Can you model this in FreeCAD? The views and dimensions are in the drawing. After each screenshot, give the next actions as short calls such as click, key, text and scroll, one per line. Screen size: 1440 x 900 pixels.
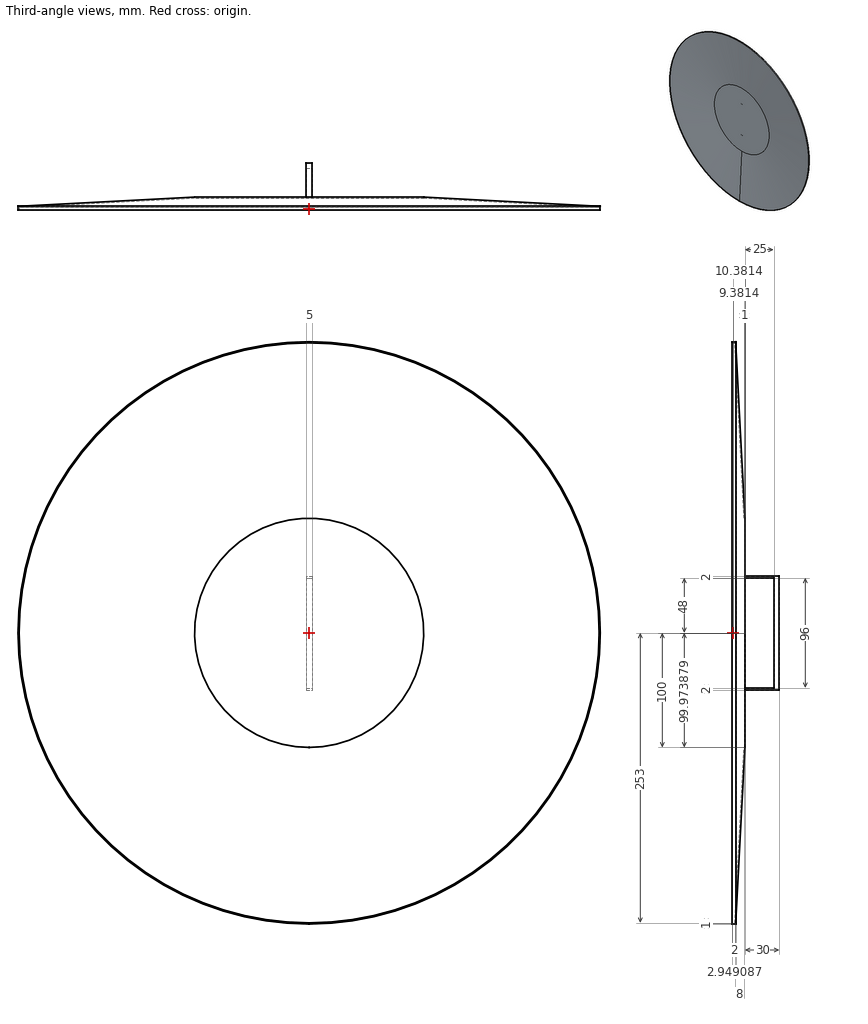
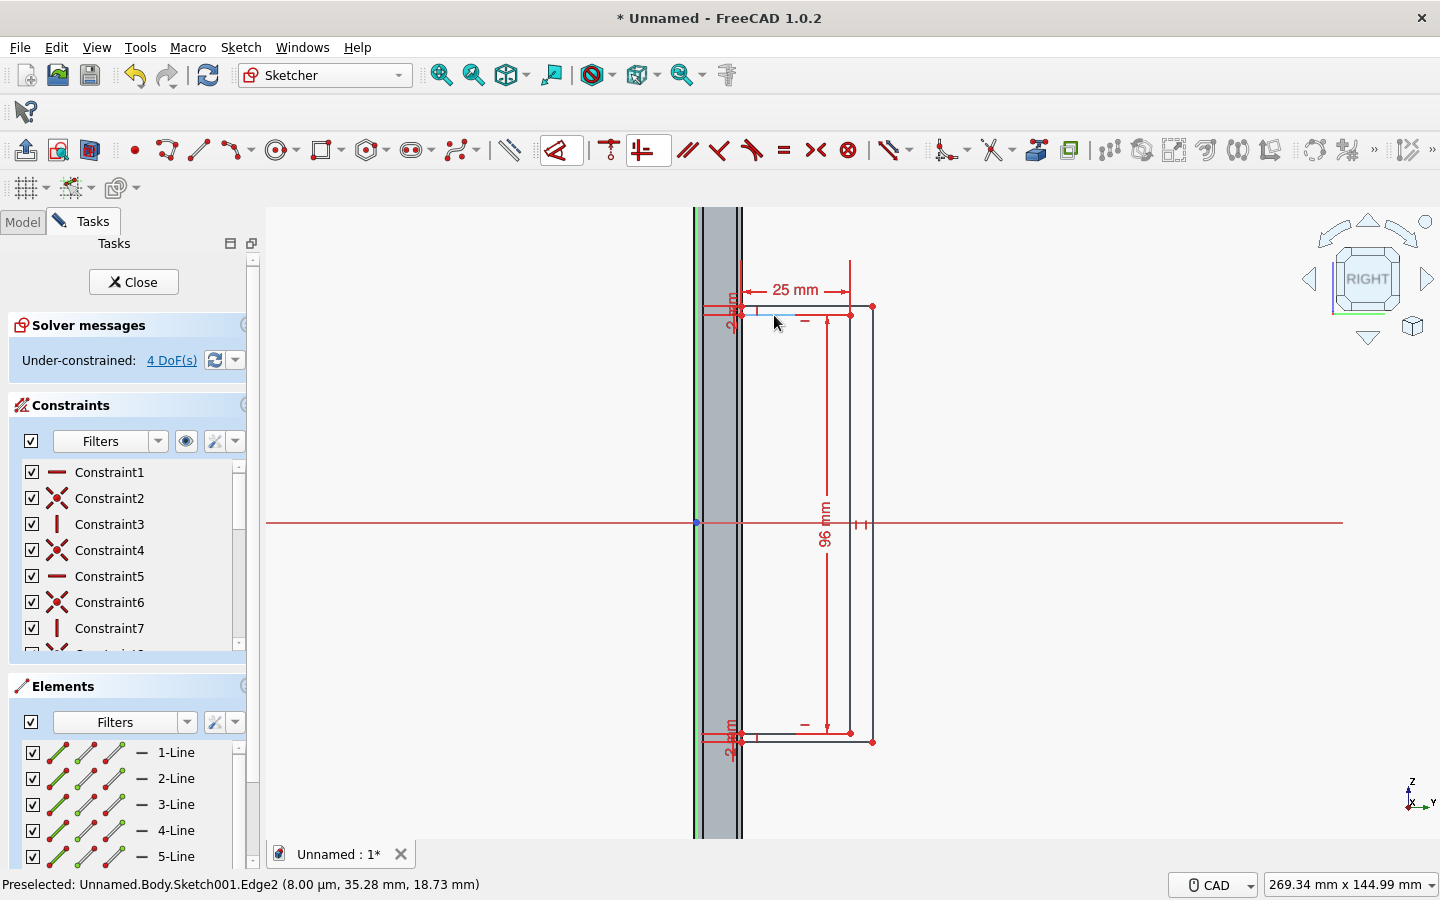
scroll(818, 734, up, 3)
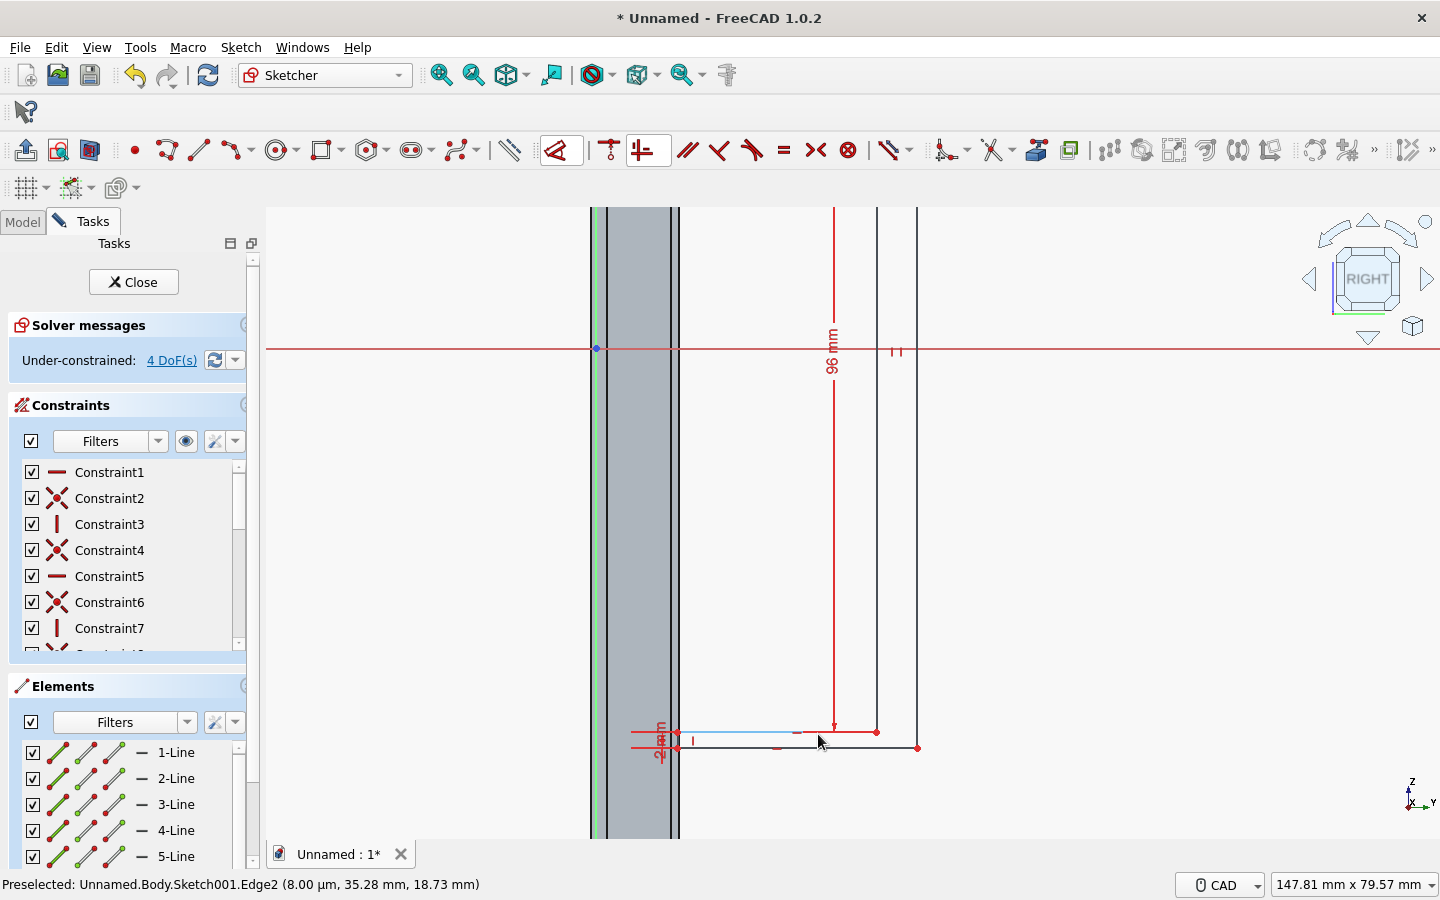
click(817, 732)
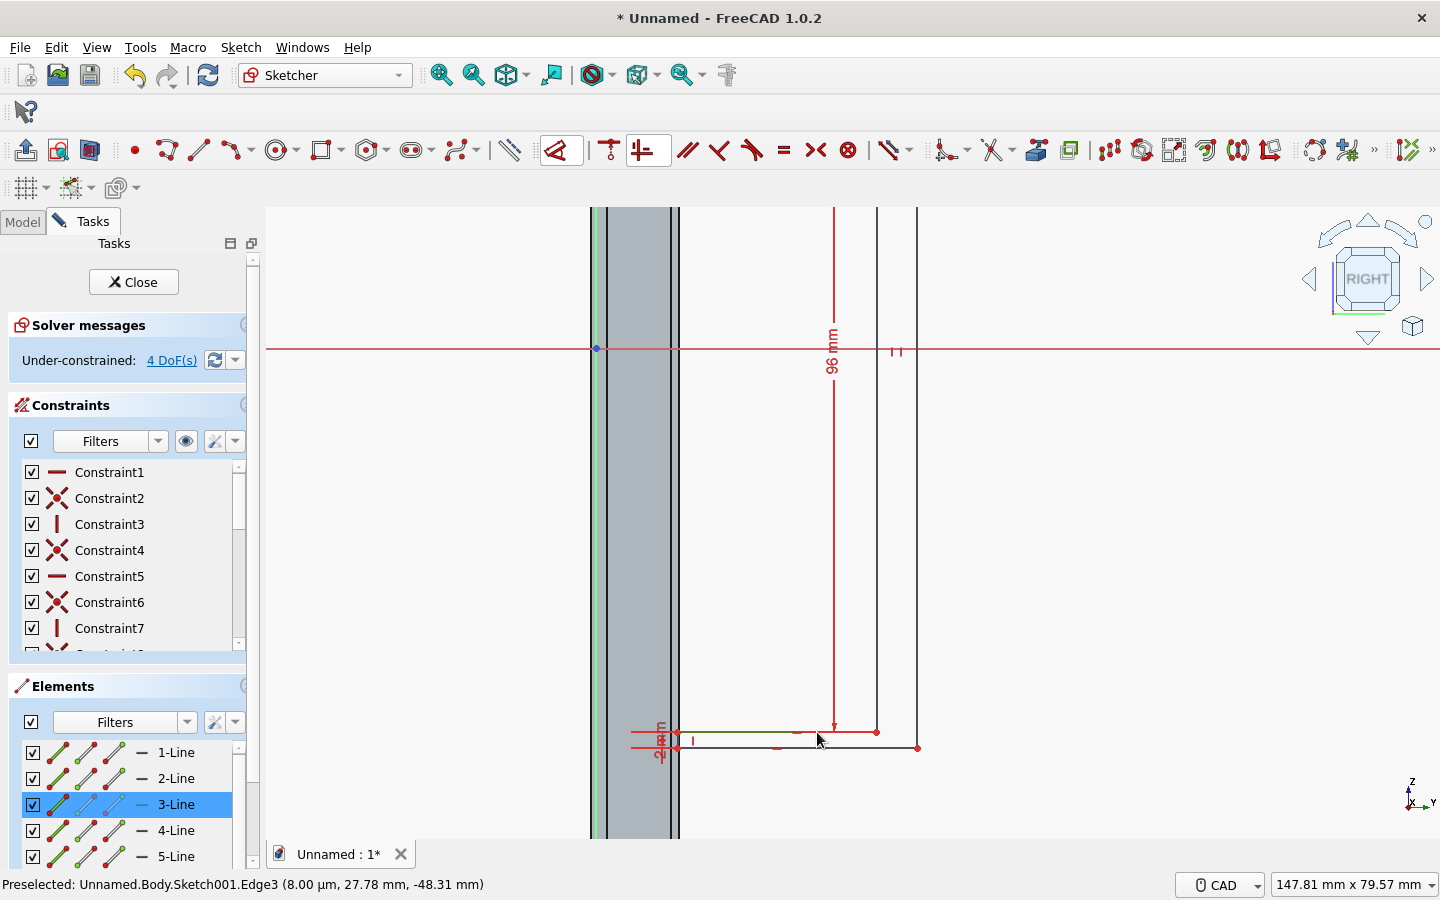
key(l)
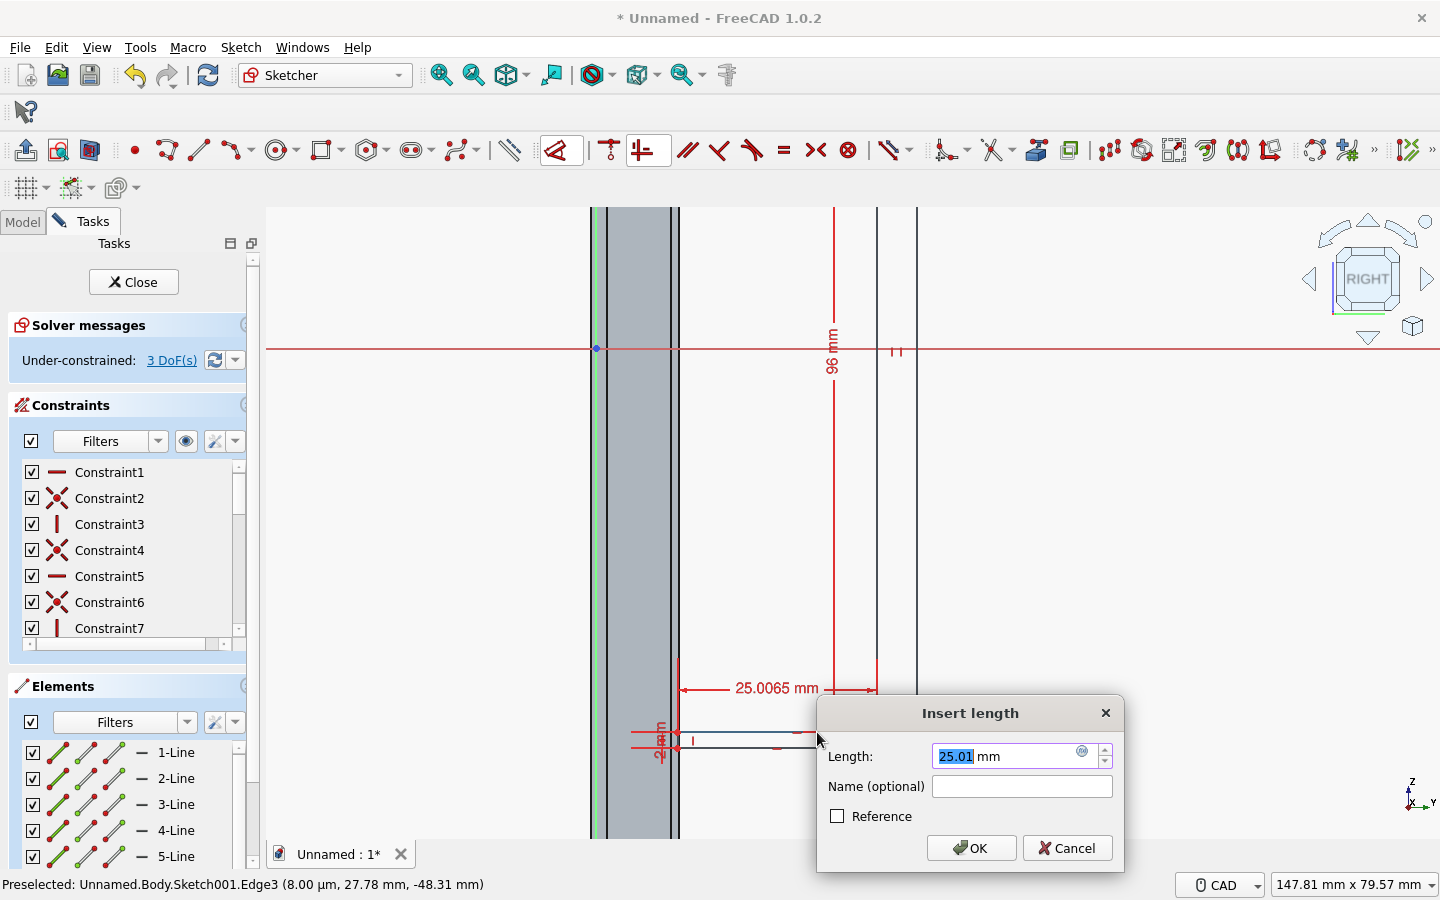
text(25)
key(Return)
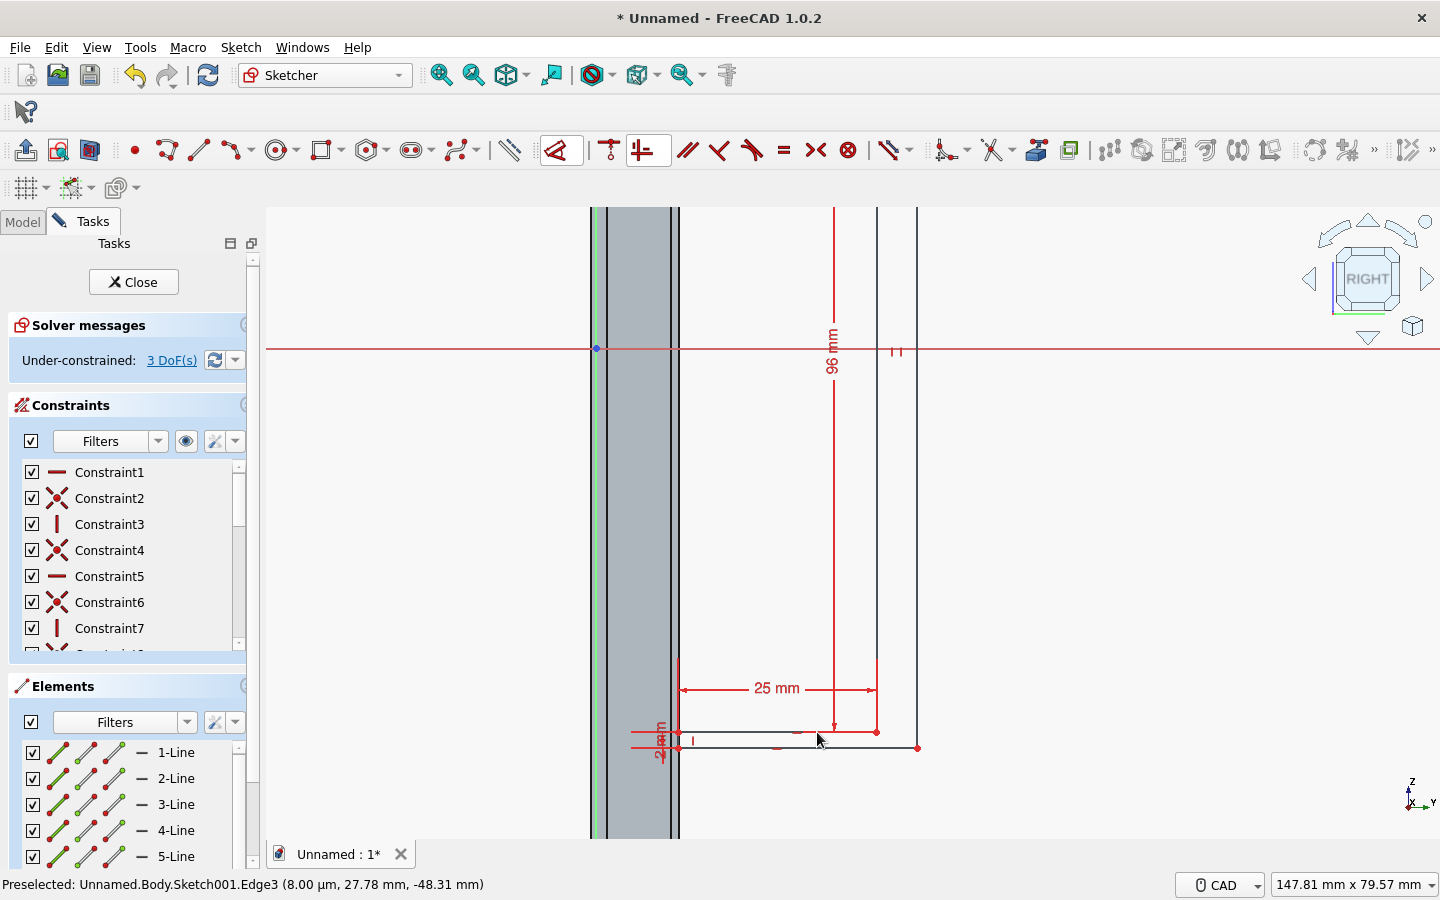
click(750, 748)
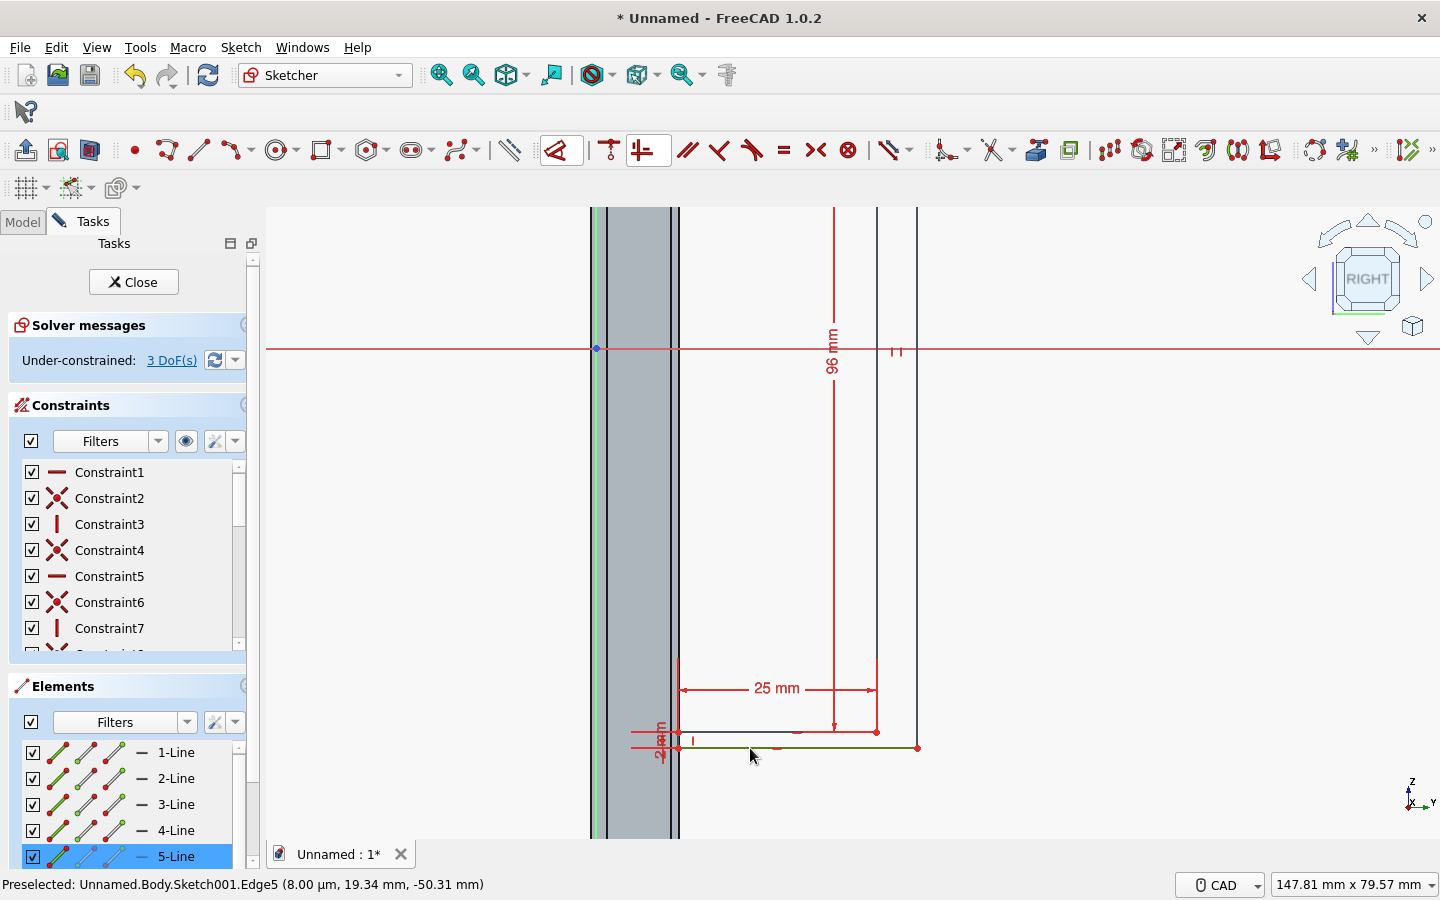
click(578, 150)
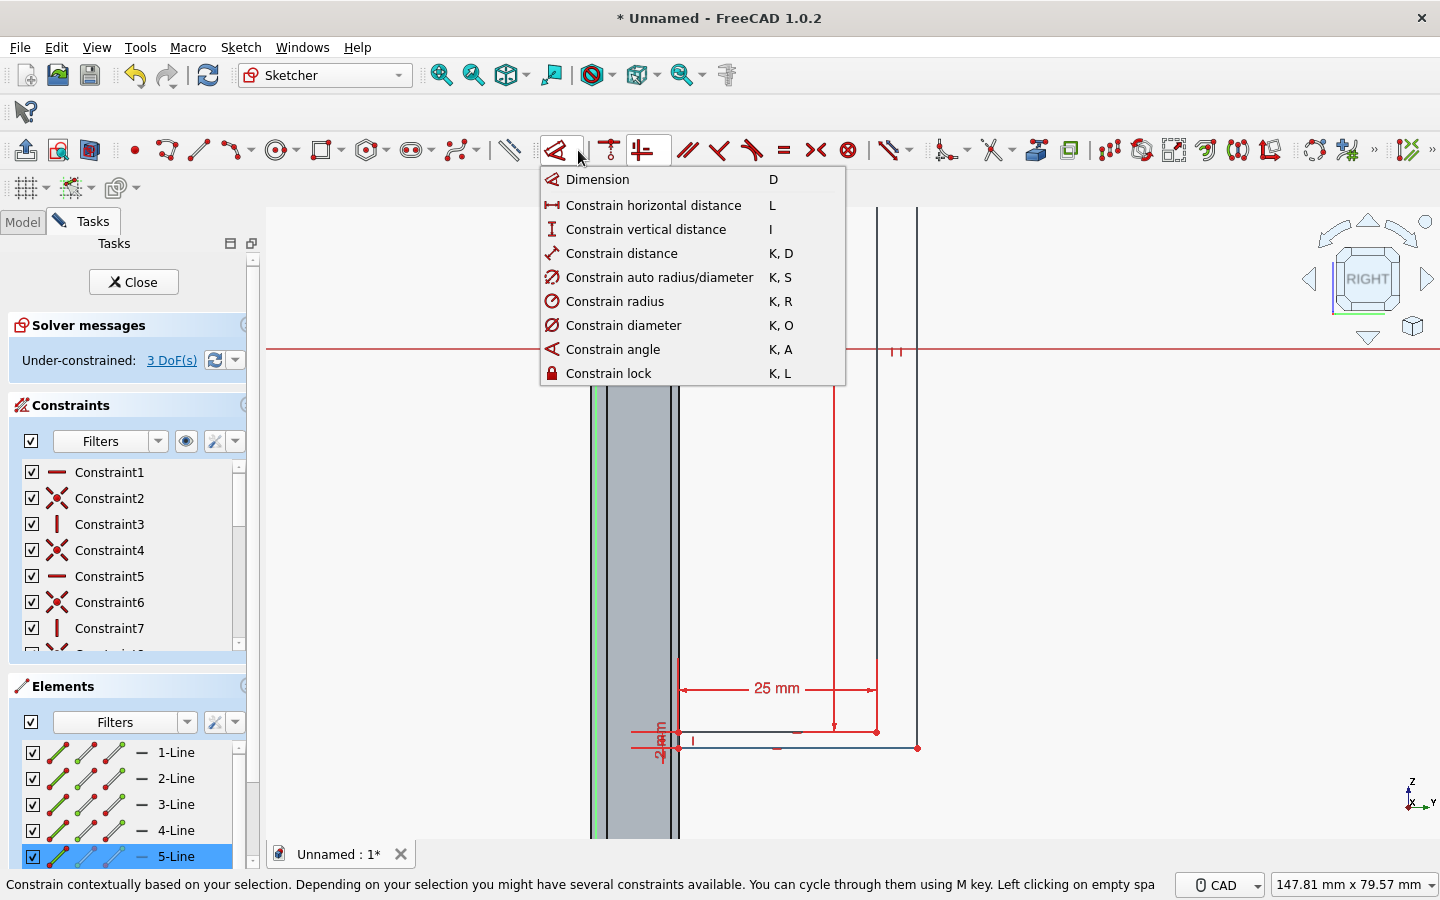
click(693, 205)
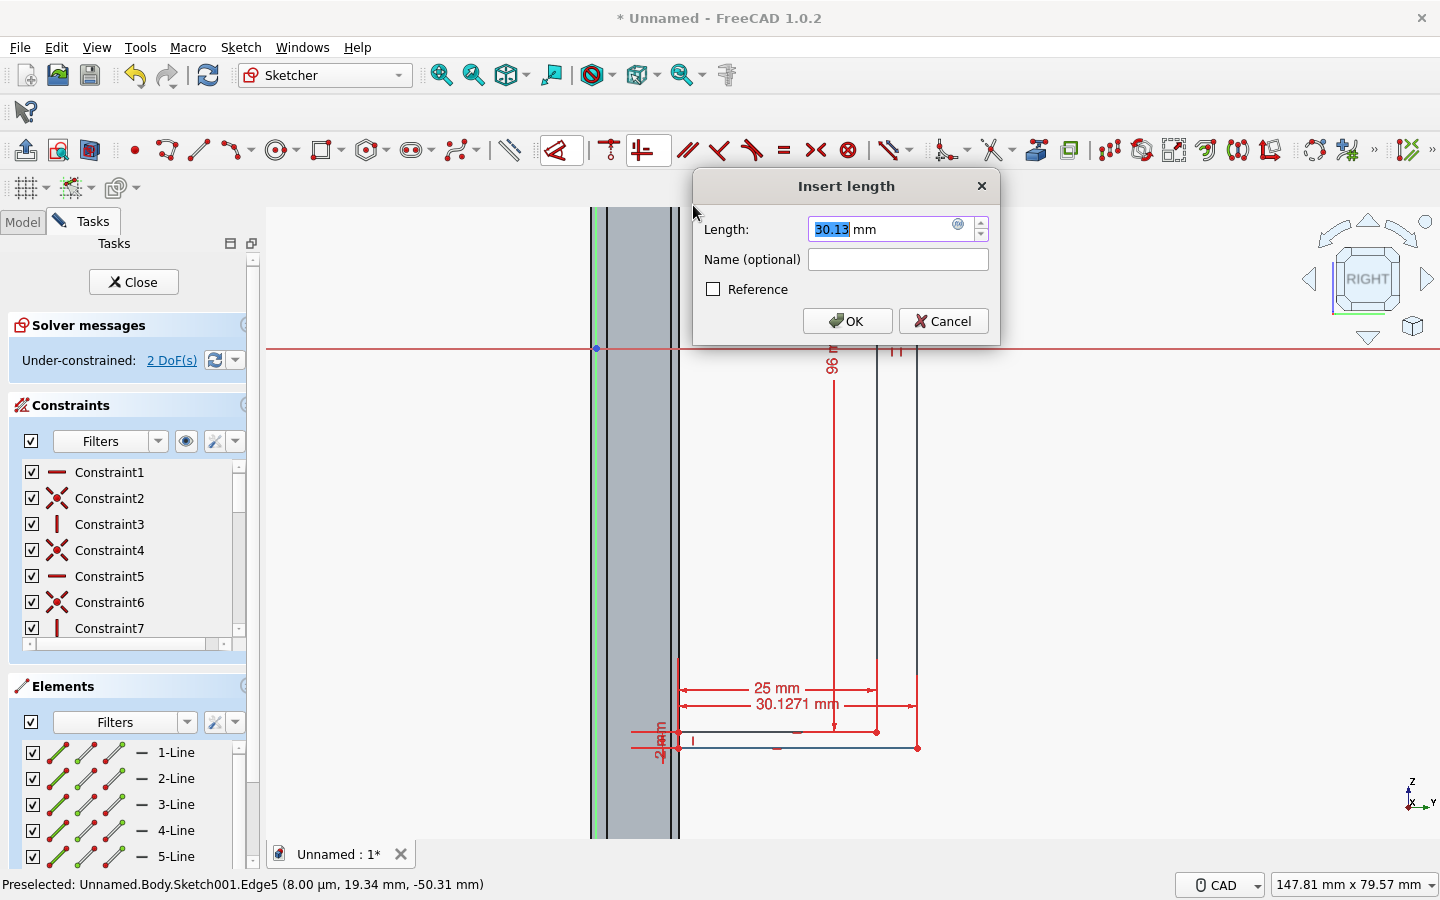
text(30)
key(Return)